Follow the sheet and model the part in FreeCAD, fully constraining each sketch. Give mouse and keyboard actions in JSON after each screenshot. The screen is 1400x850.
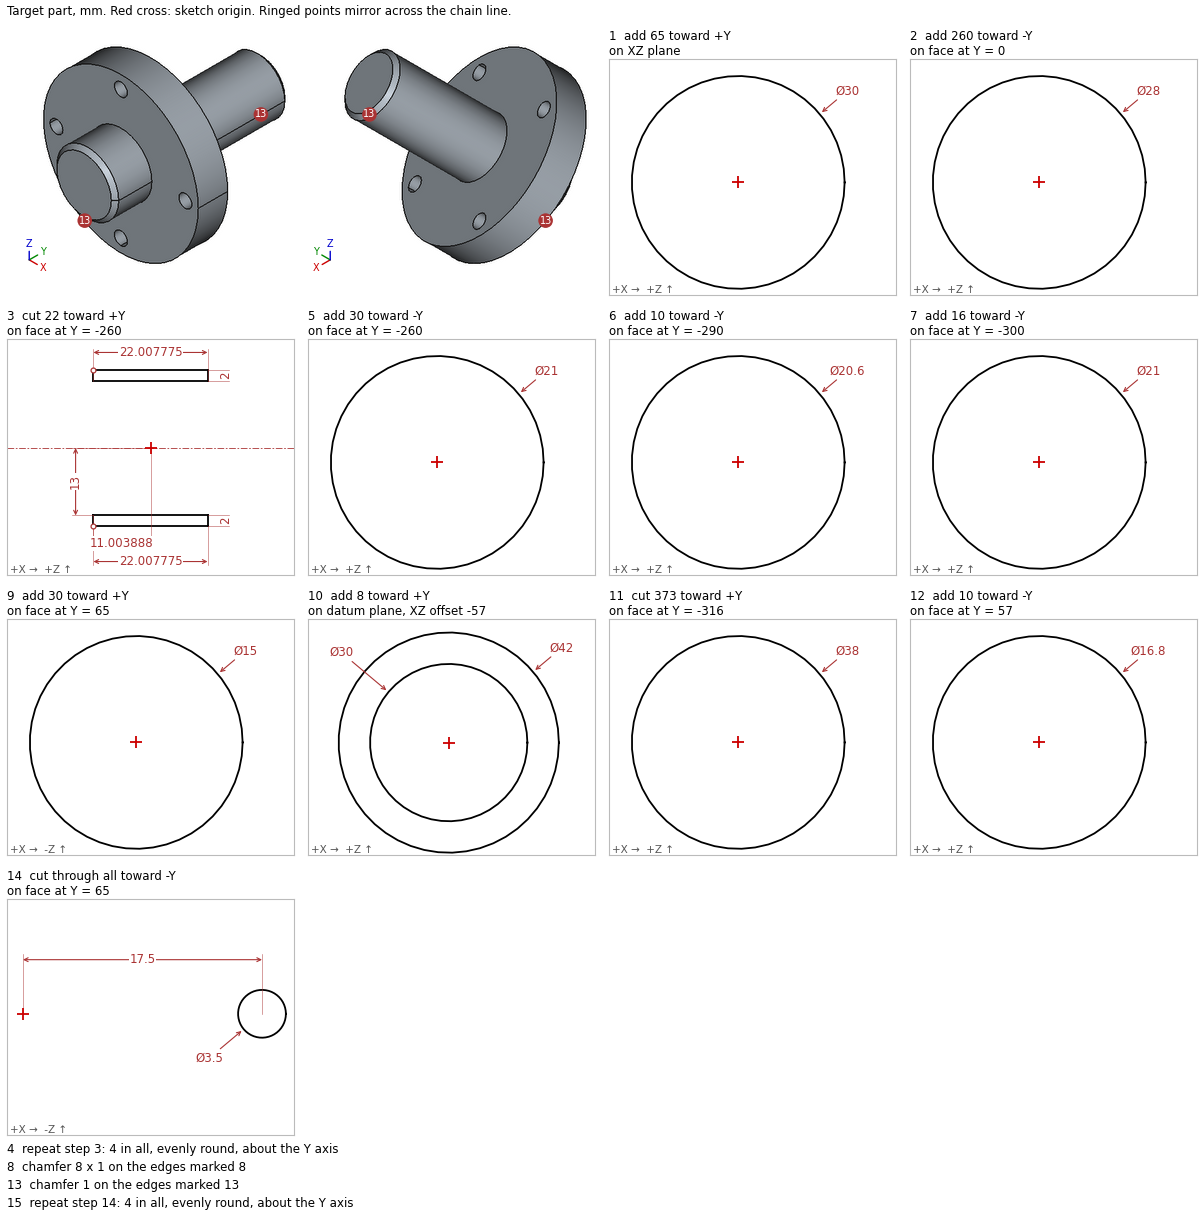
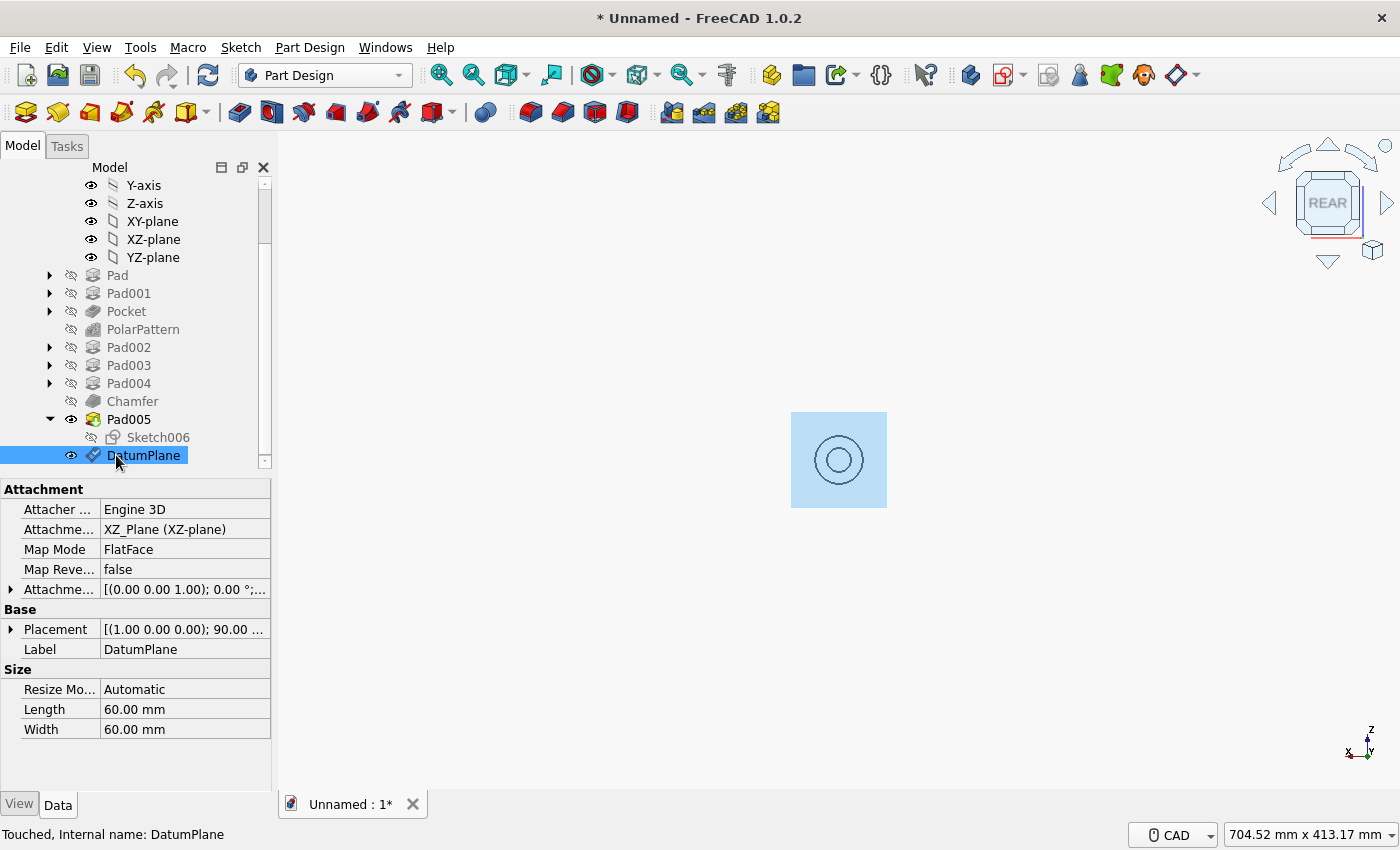
{"action": "left_click", "coordinate": [1004, 76]}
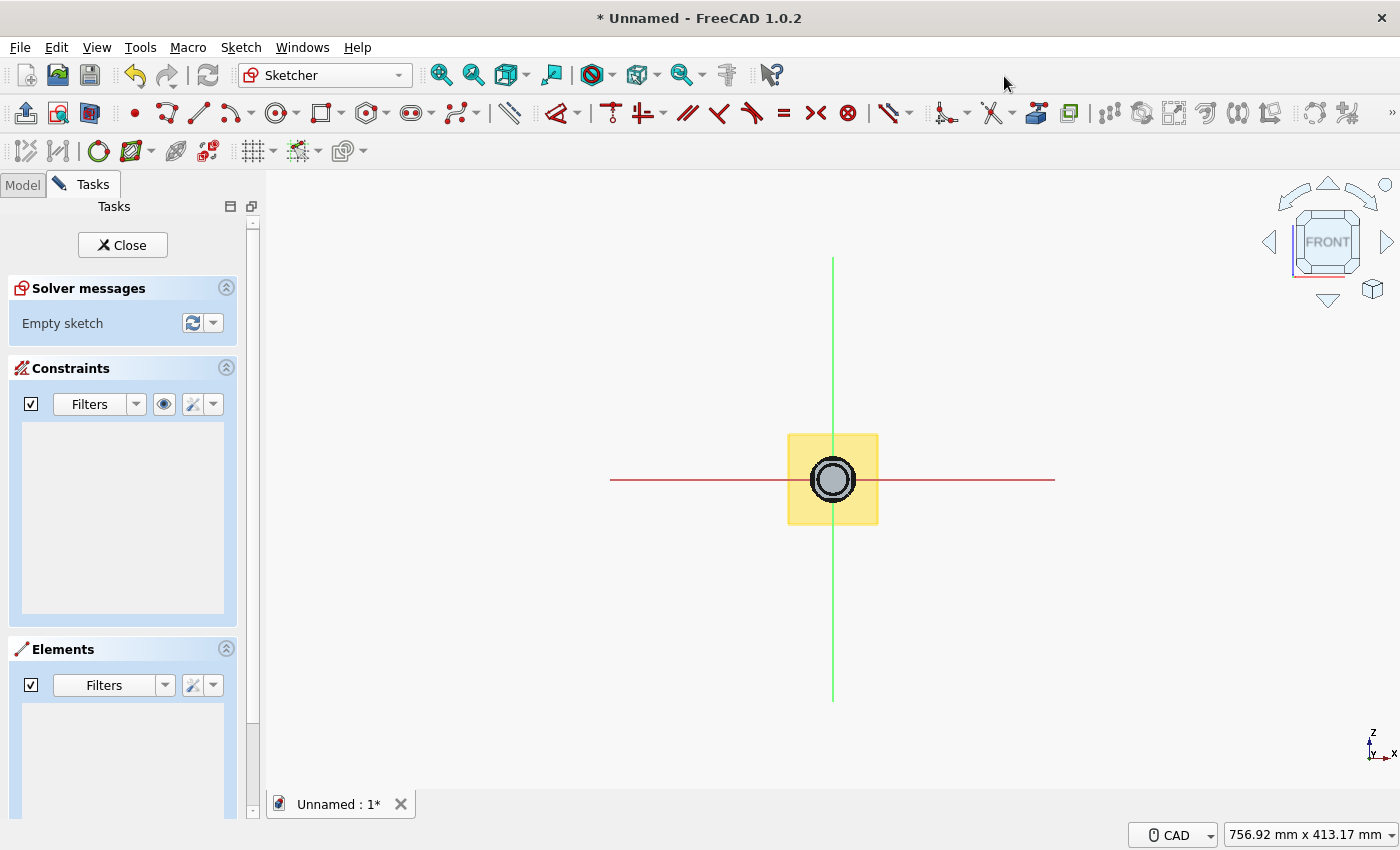
{"action": "left_click", "coordinate": [90, 114]}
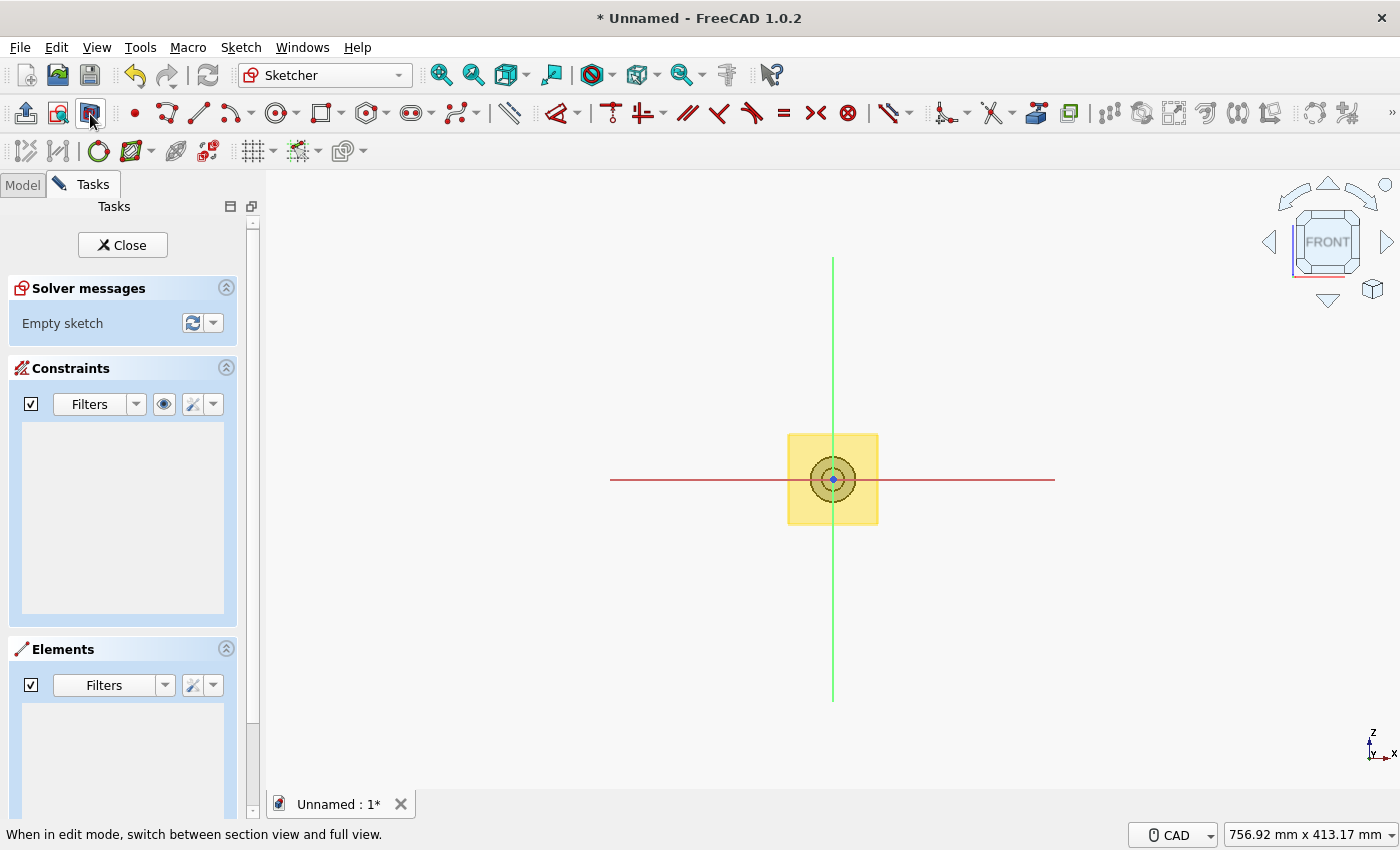
{"action": "scroll", "coordinate": [847, 479], "scroll_direction": "up", "scroll_amount": 9}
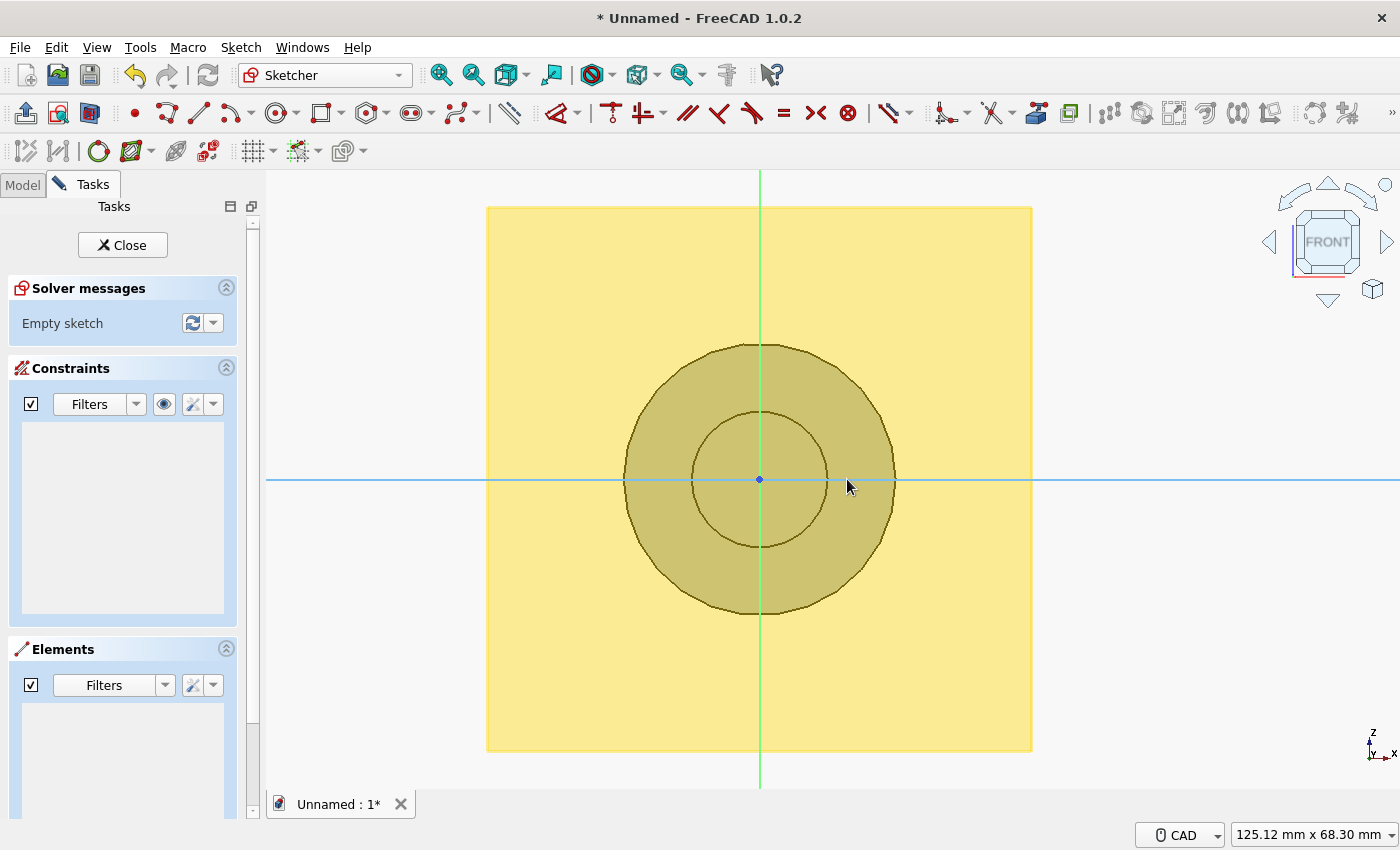
{"action": "left_click", "coordinate": [276, 114]}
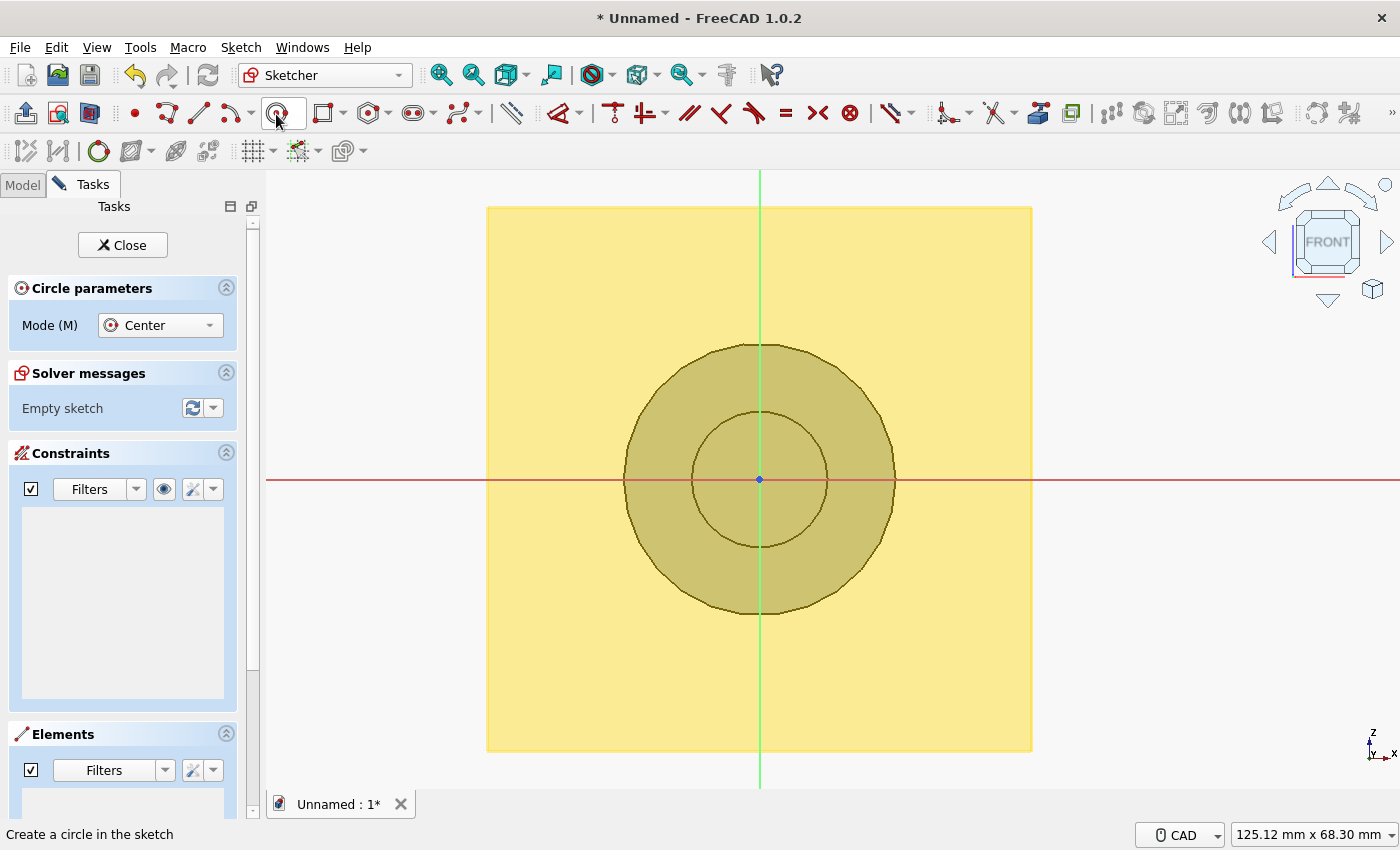
{"action": "left_click", "coordinate": [760, 479]}
{"action": "mouse_move", "coordinate": [894, 345]}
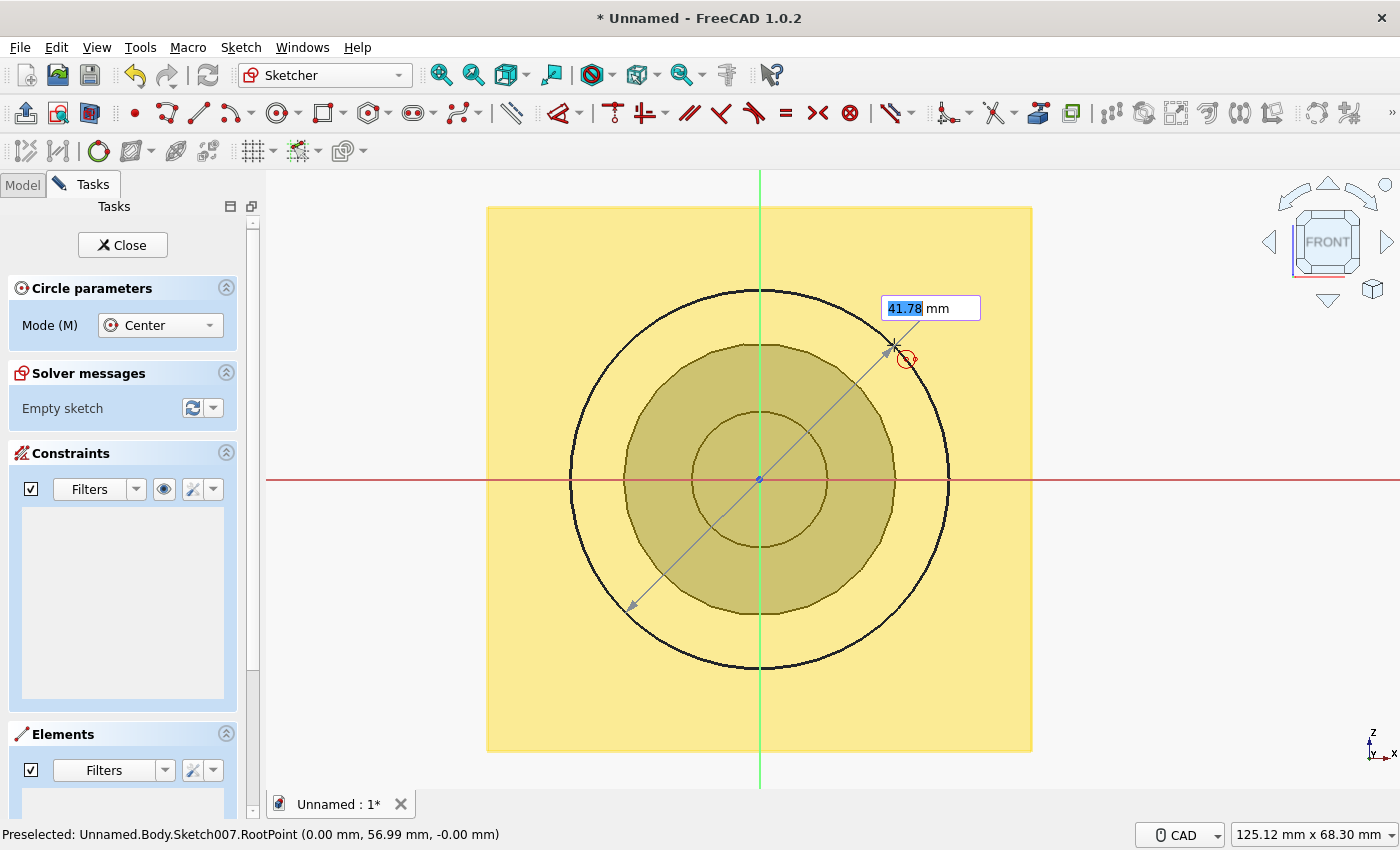
{"action": "type", "text": "42"}
{"action": "key", "text": "Return"}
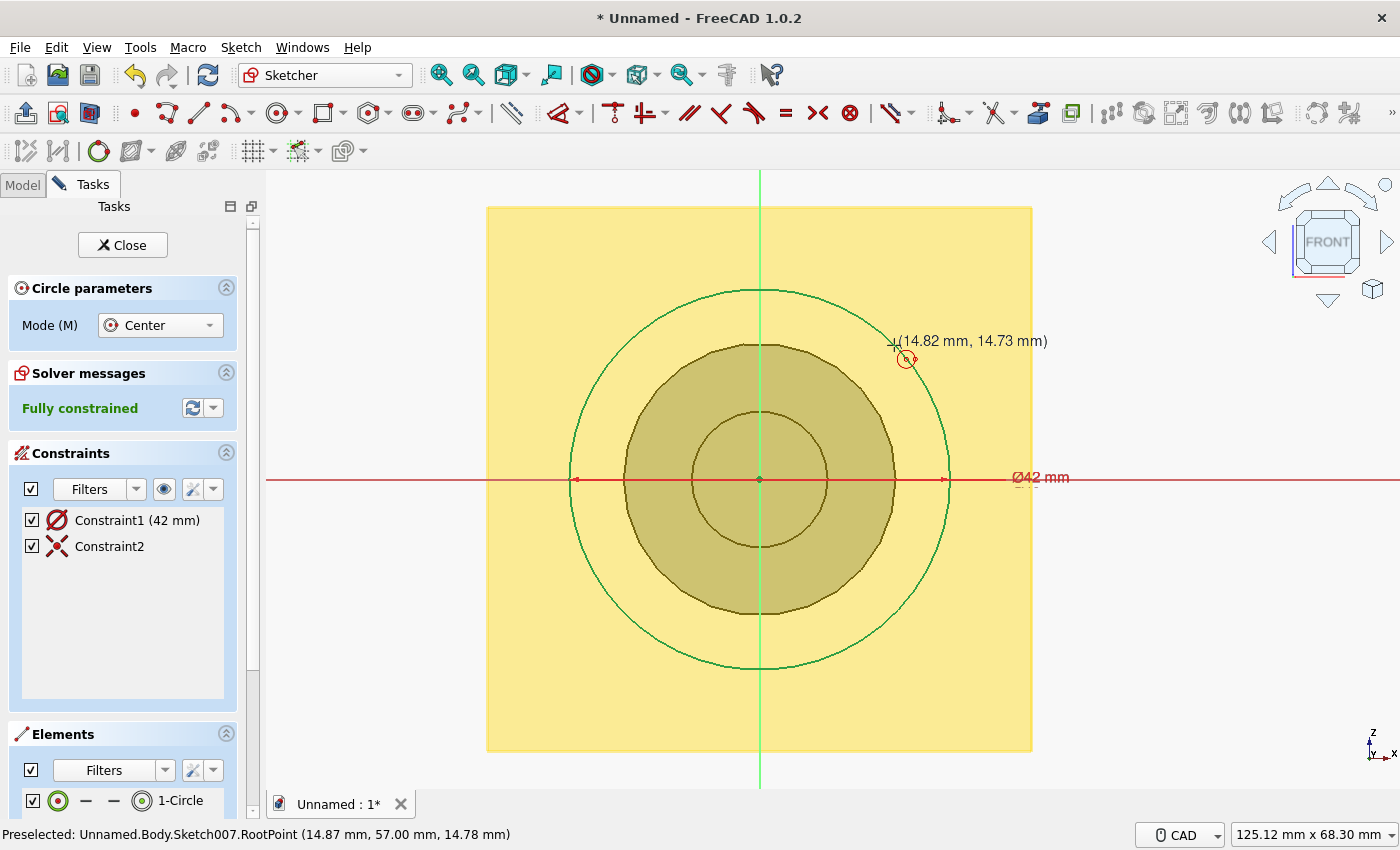
{"action": "left_click", "coordinate": [760, 479]}
{"action": "mouse_move", "coordinate": [856, 383]}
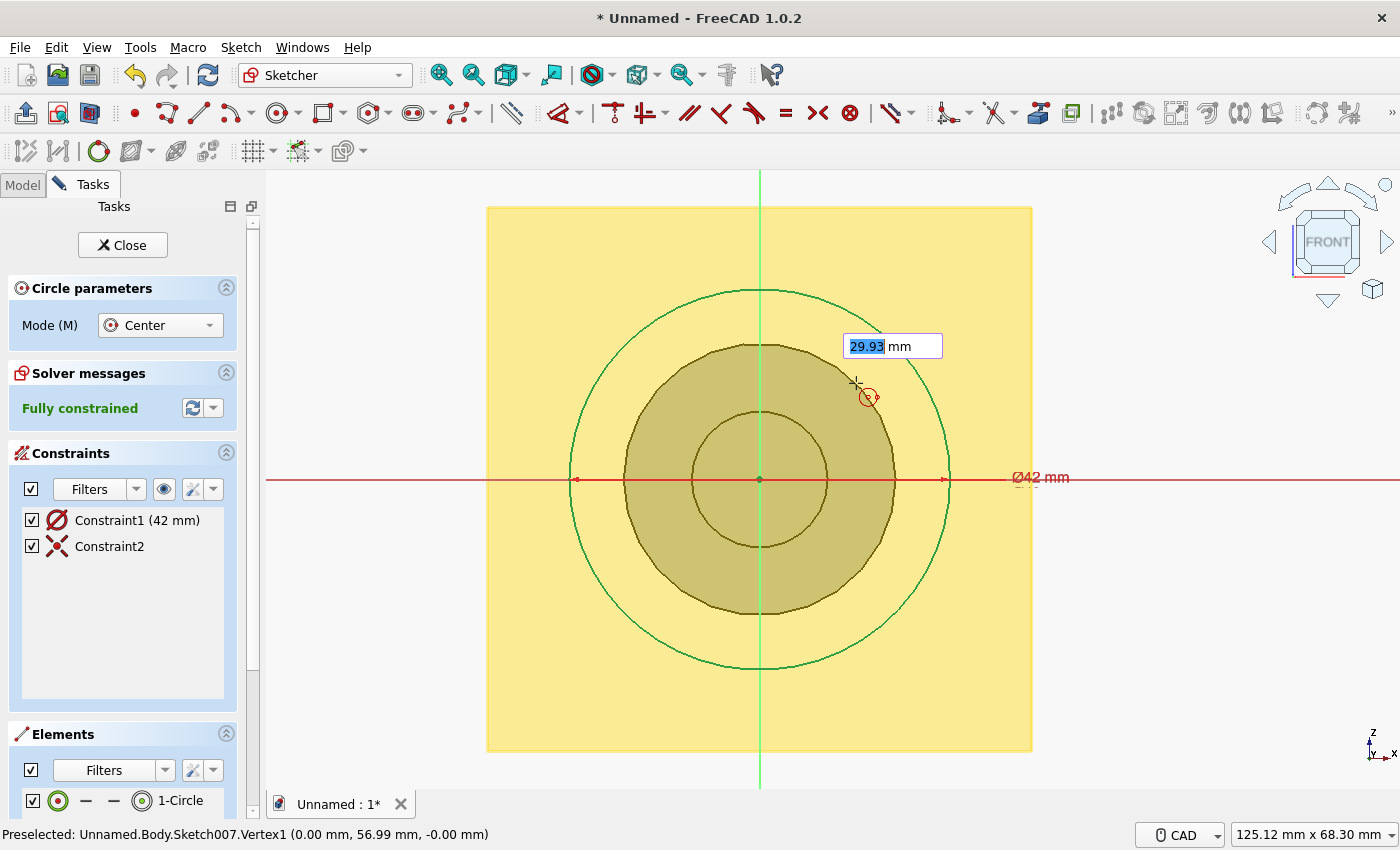
{"action": "type", "text": "30"}
{"action": "key", "text": "Return"}
{"action": "key", "text": "Escape"}